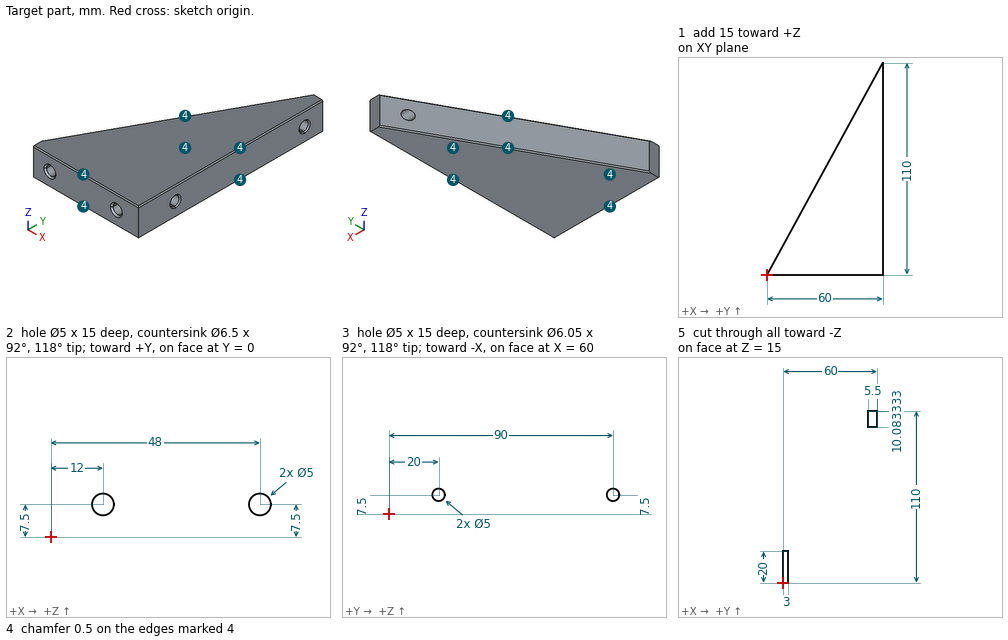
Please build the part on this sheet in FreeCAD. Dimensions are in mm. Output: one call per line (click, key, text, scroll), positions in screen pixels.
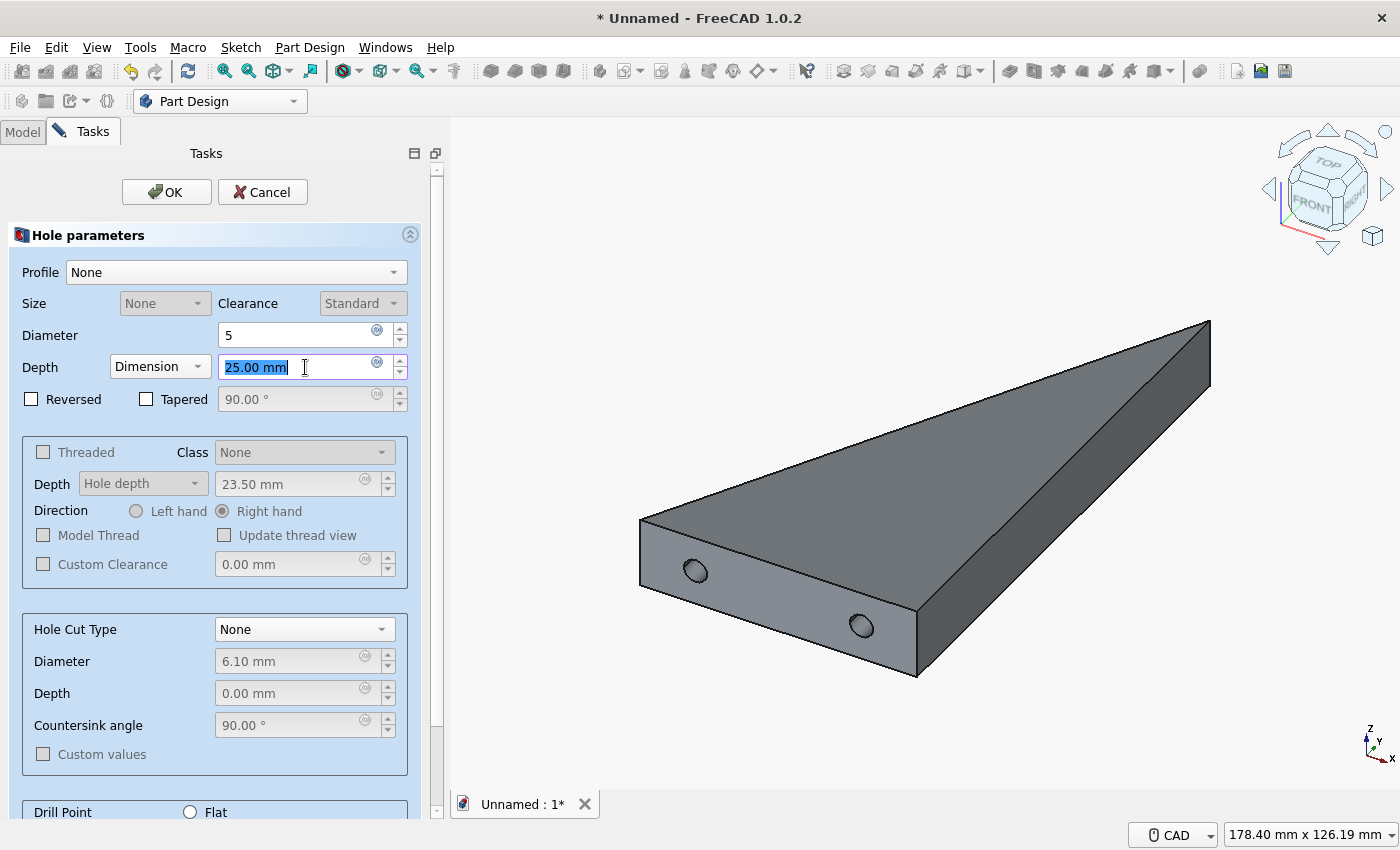
text(15)
key(Tab)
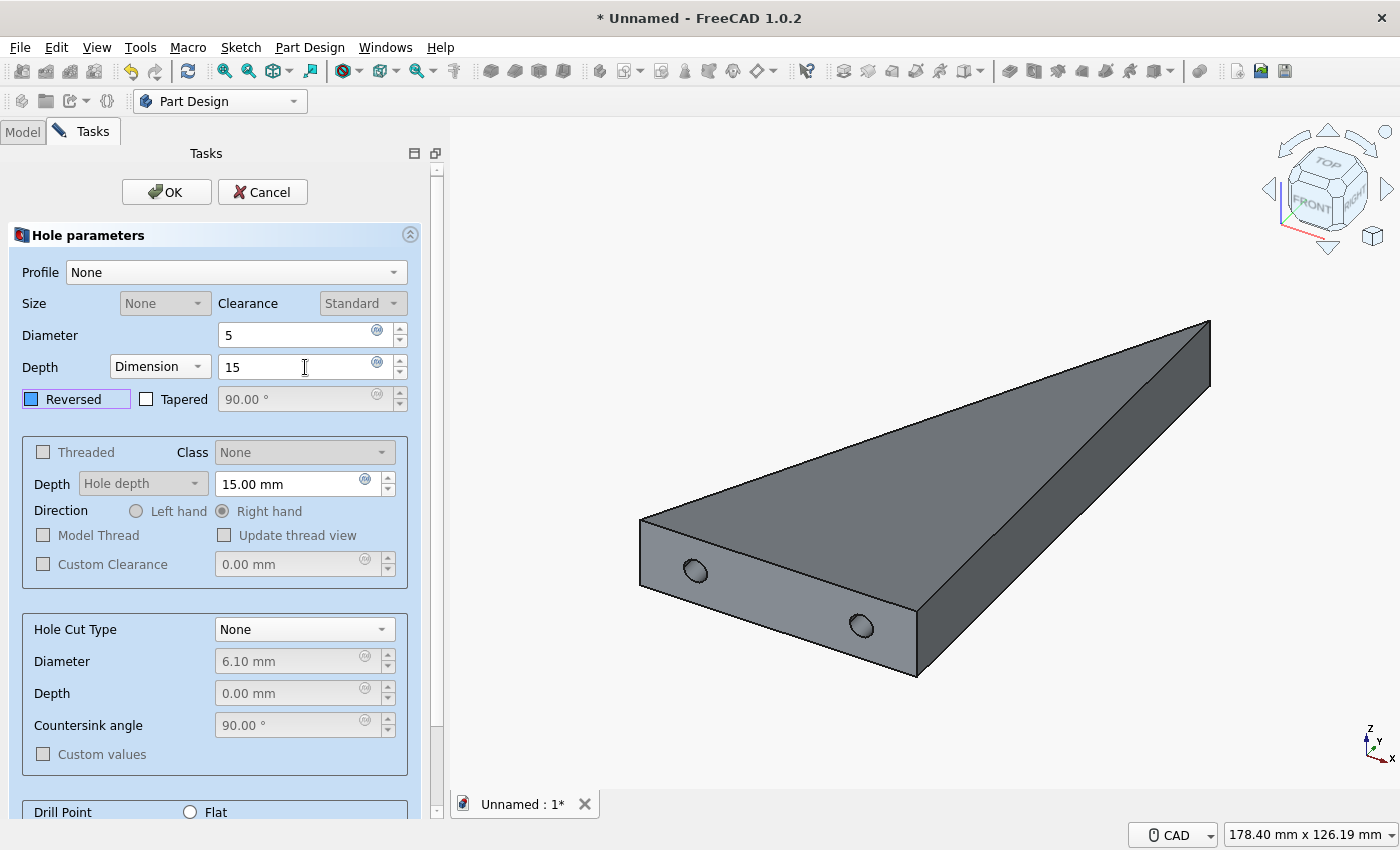
click(306, 630)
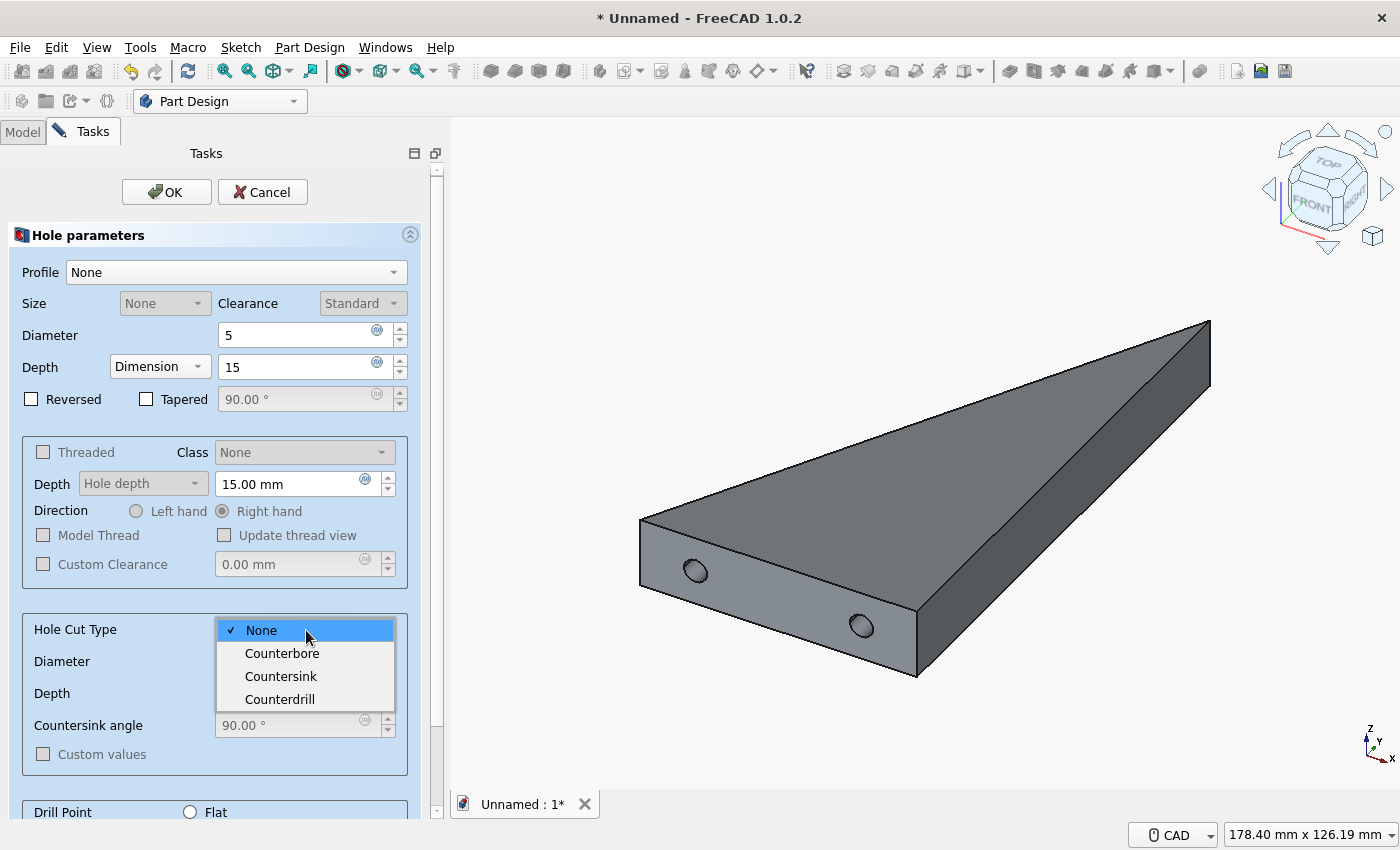
click(304, 676)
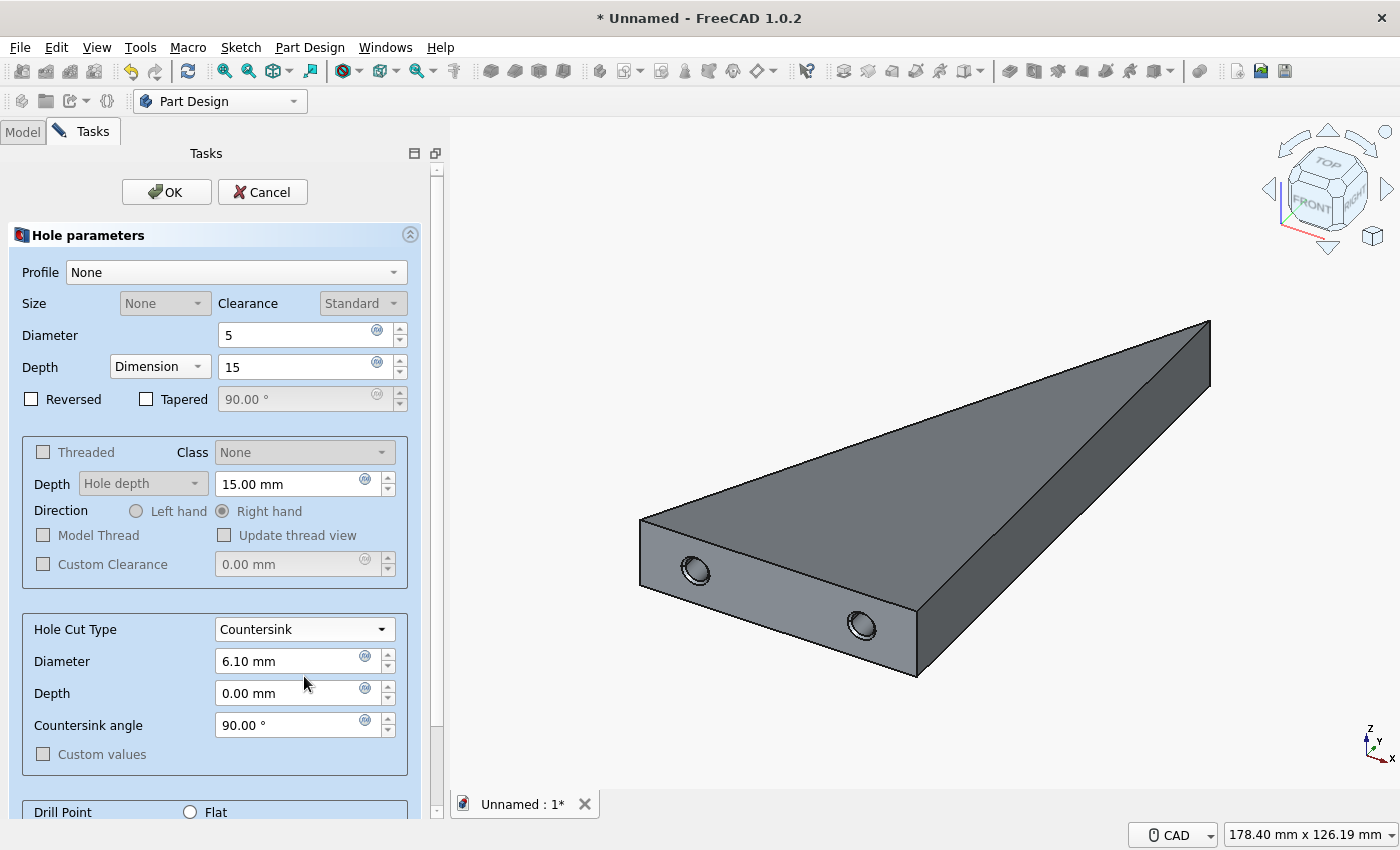
triple_click(298, 725)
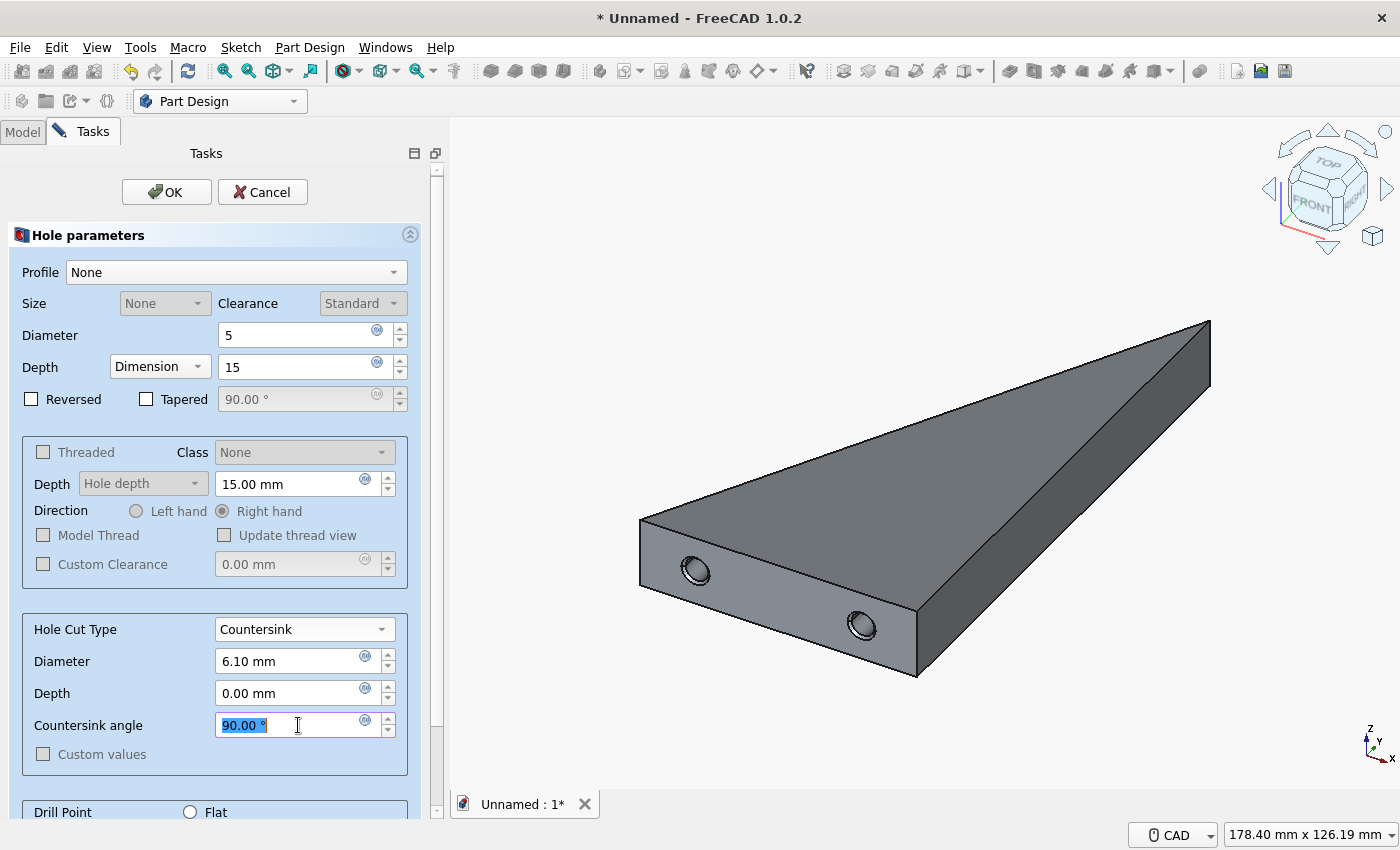
text(92)
key(Tab)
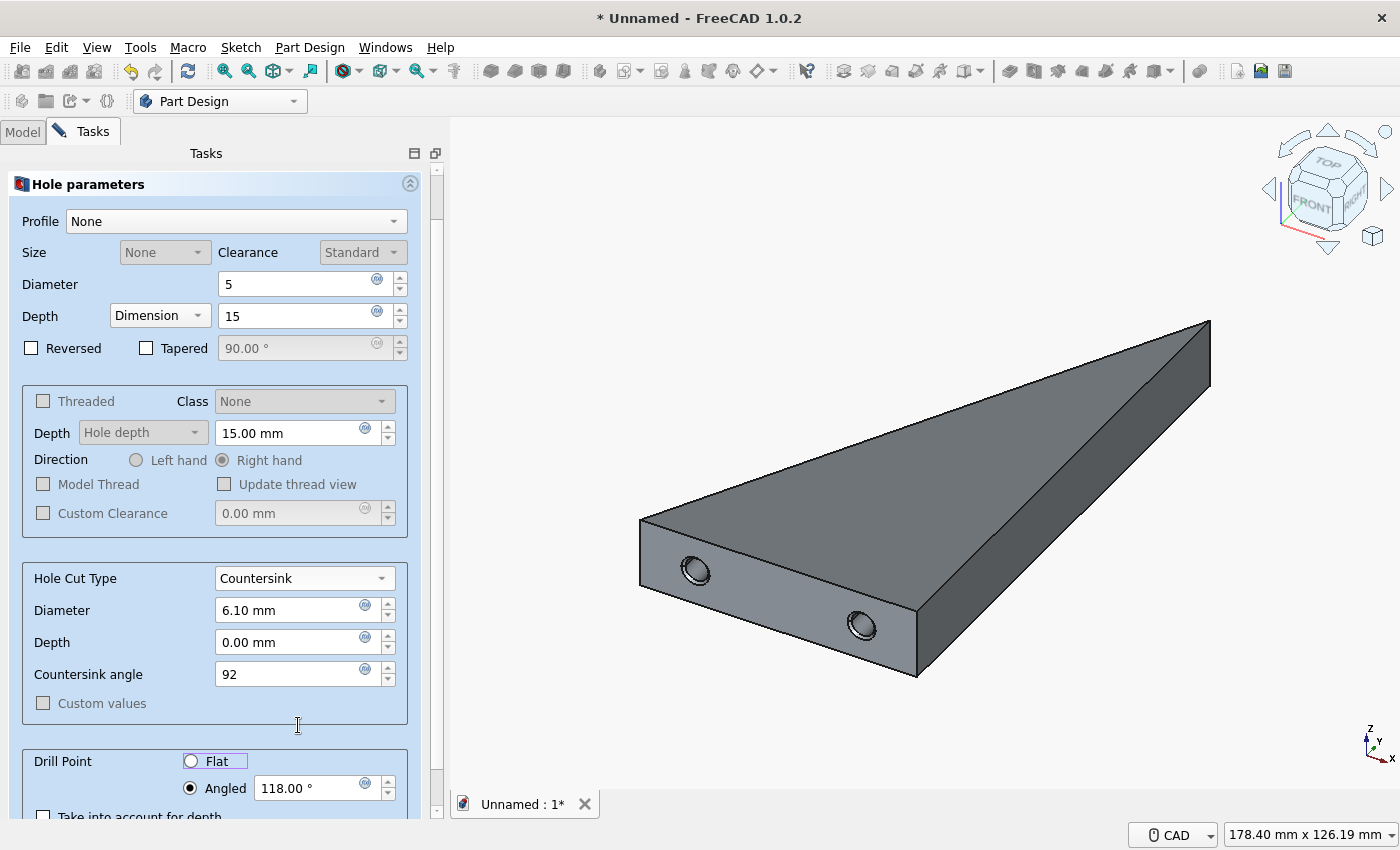
triple_click(298, 610)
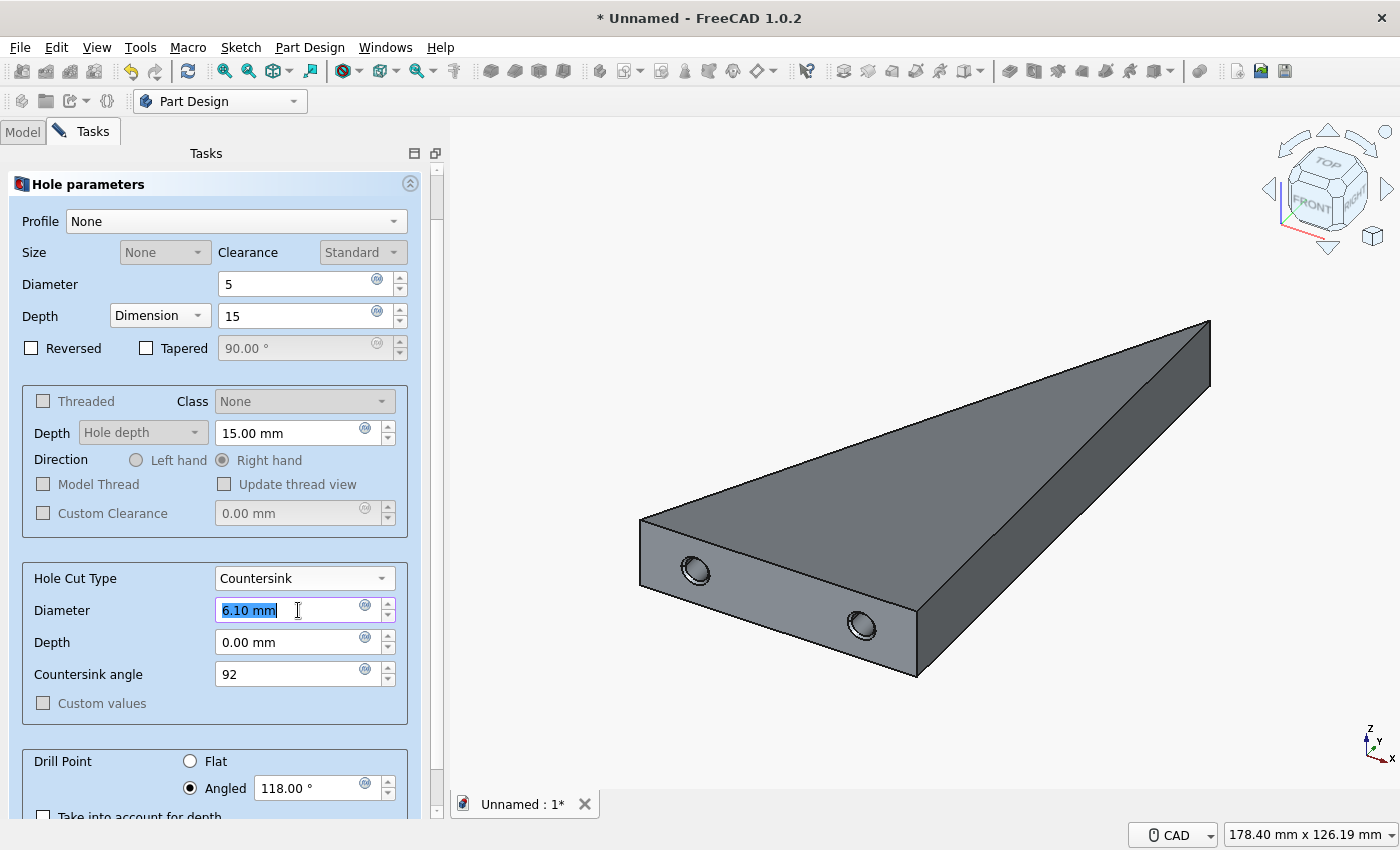
text(6.5)
key(Tab)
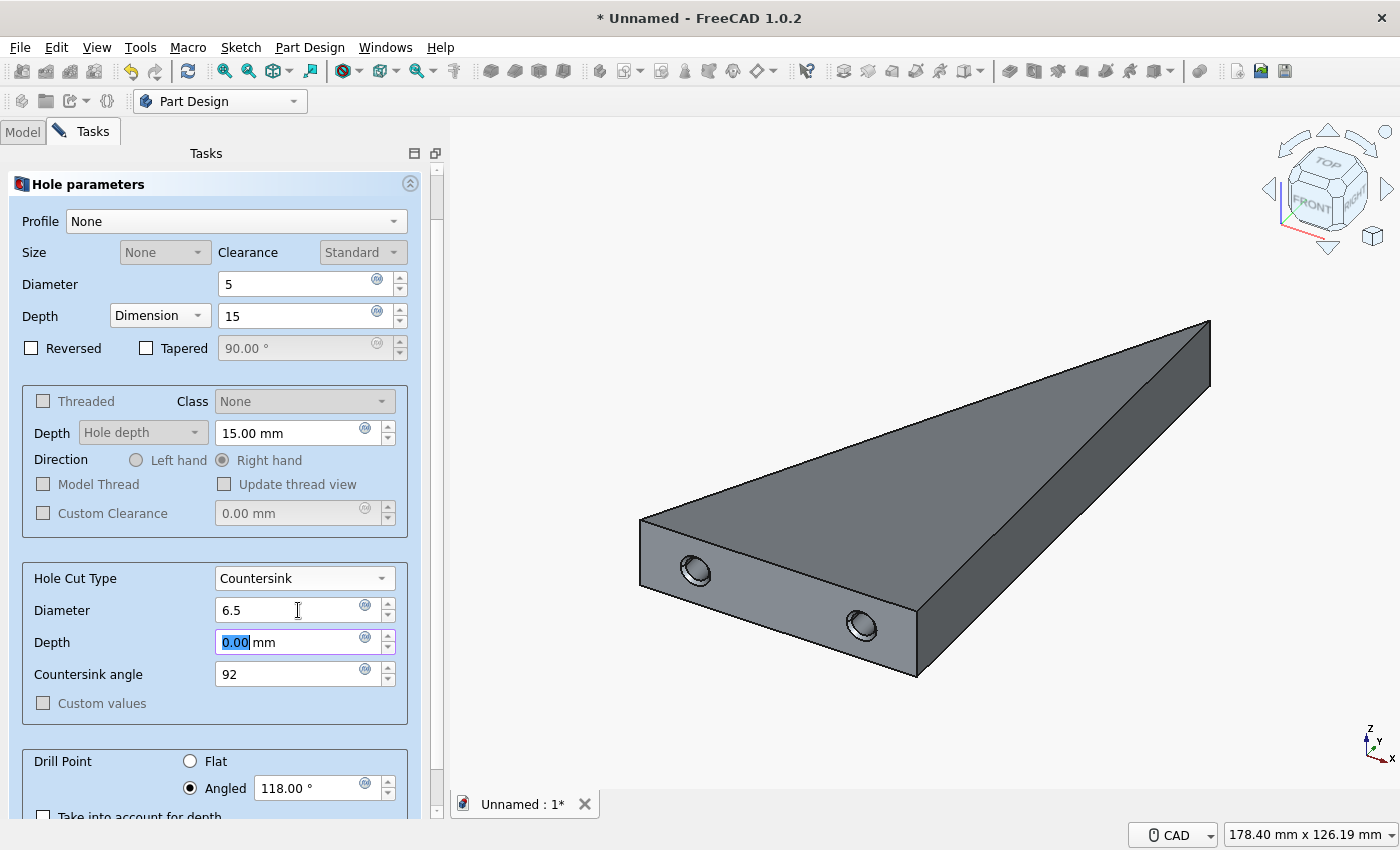
scroll(437, 490, up, 2)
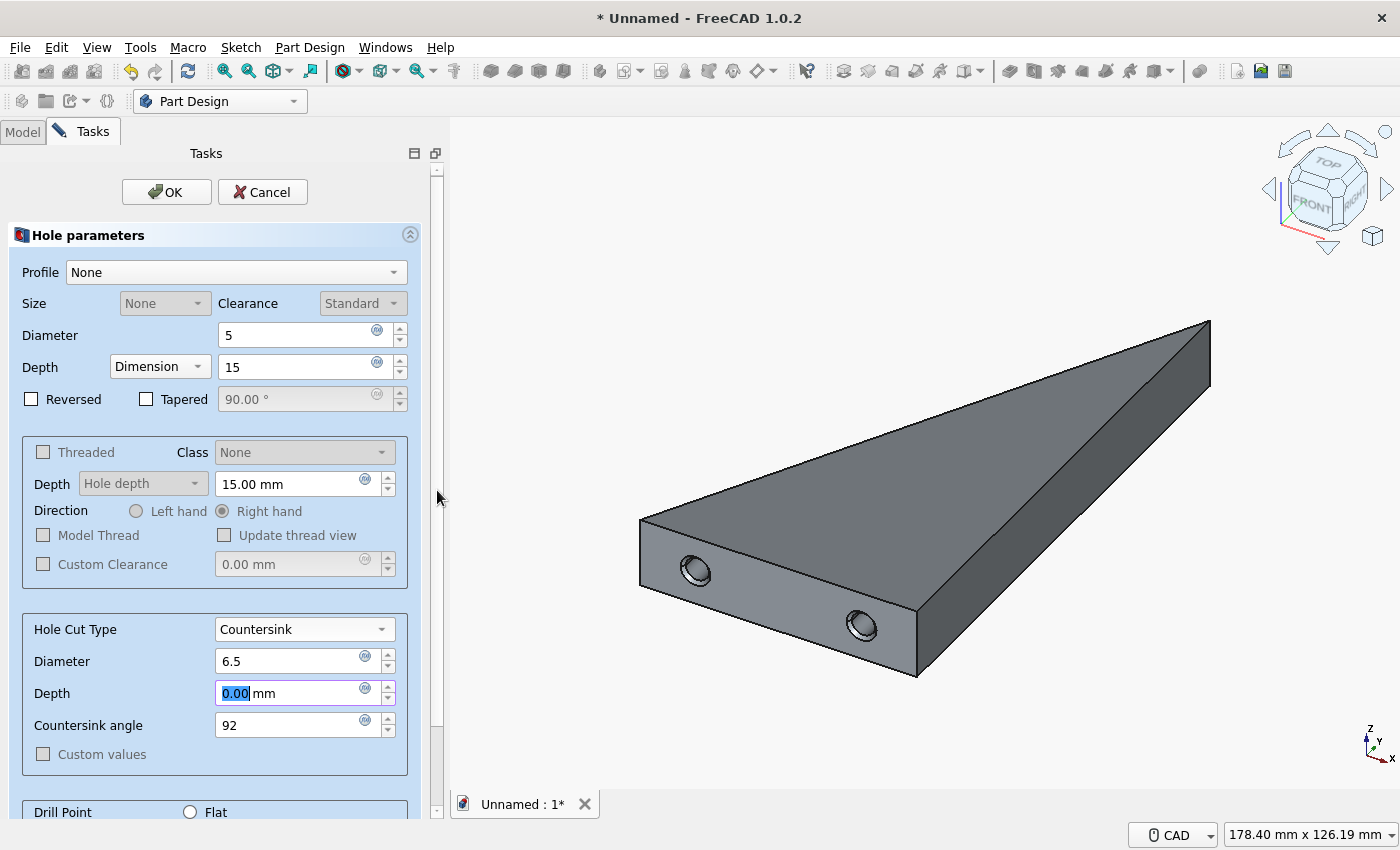
click(167, 192)